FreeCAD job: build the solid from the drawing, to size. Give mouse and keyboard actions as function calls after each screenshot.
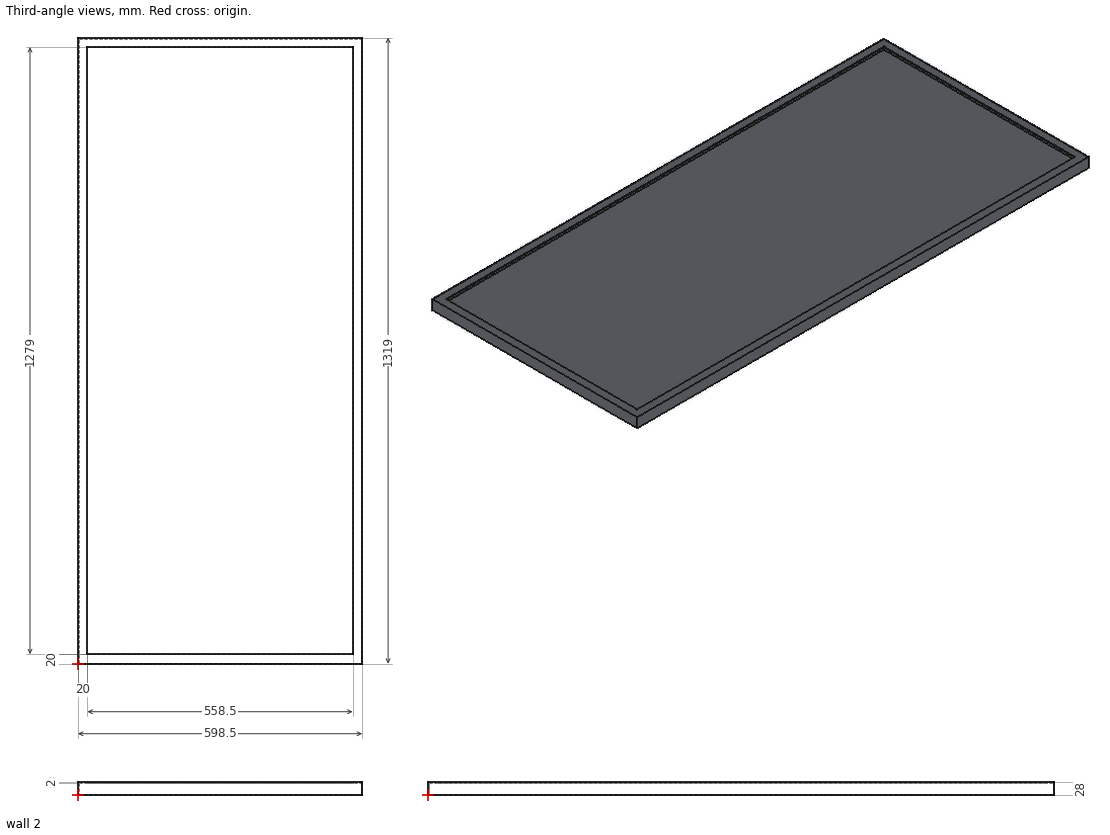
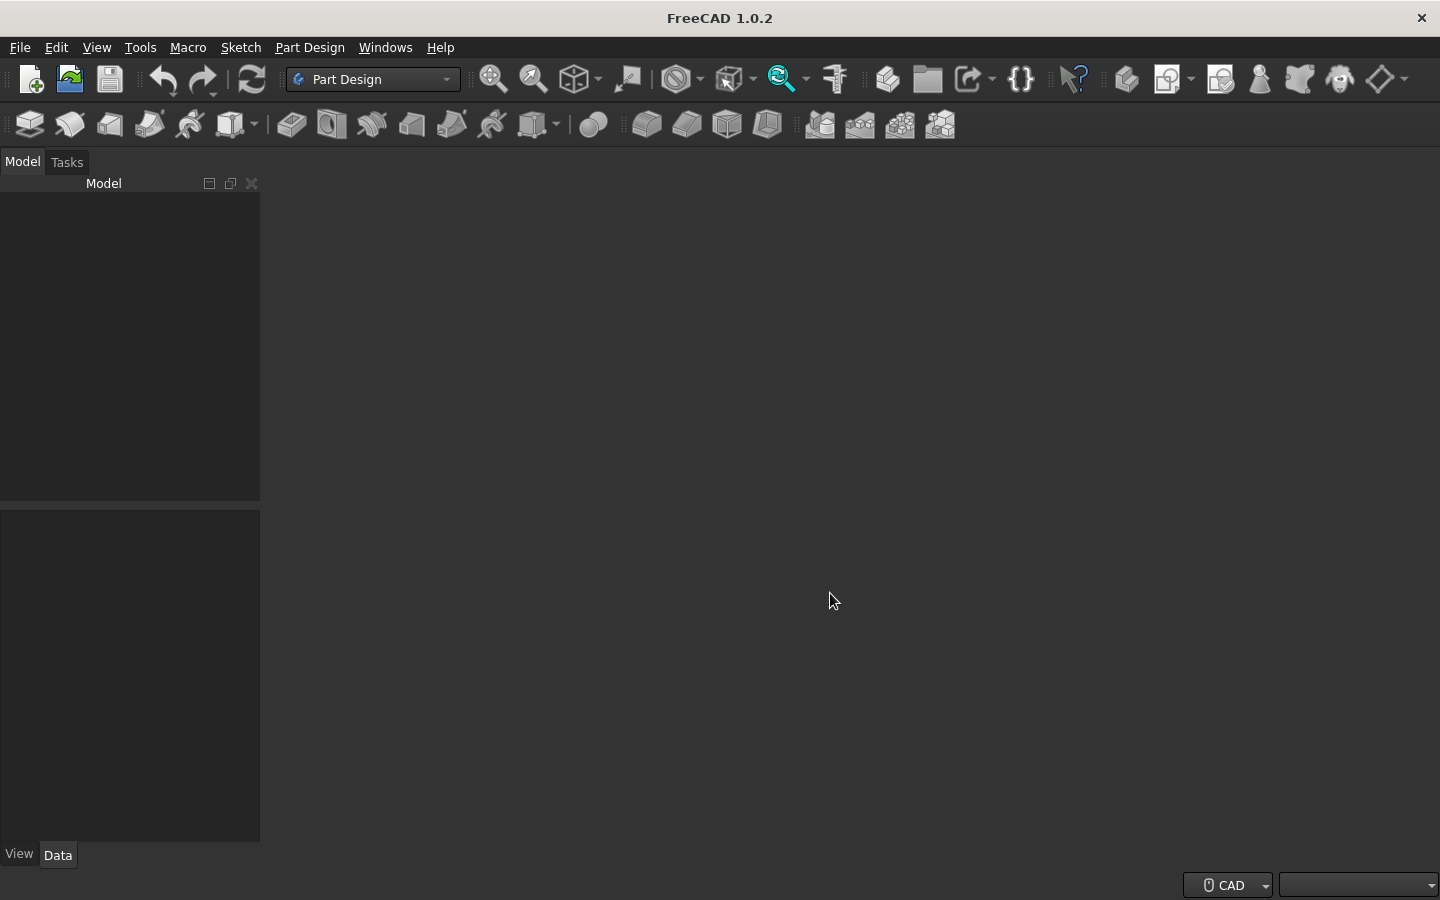
key(ctrl+n)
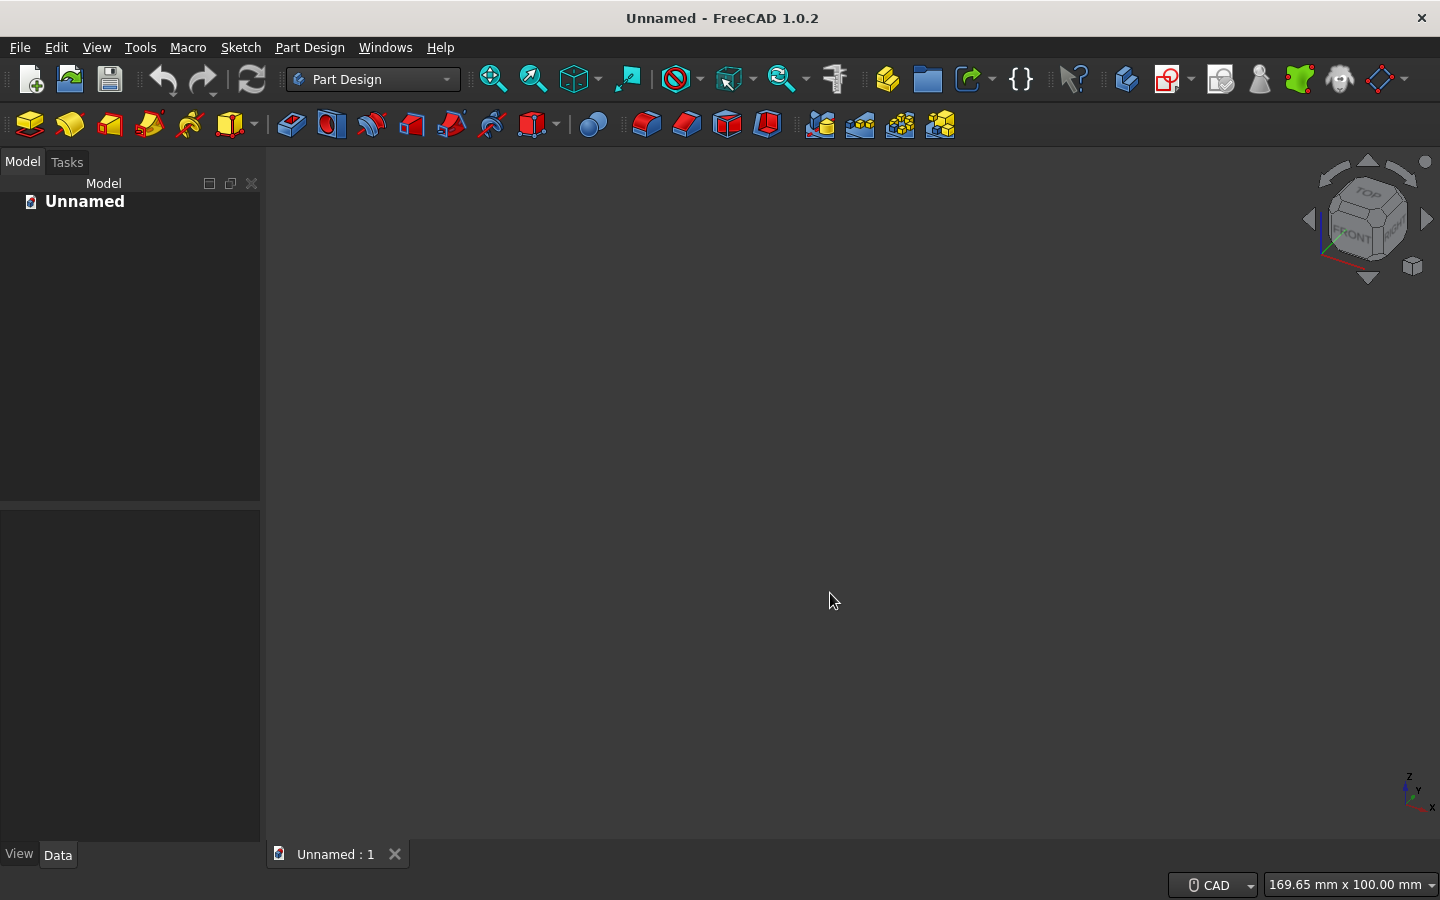
click(1168, 80)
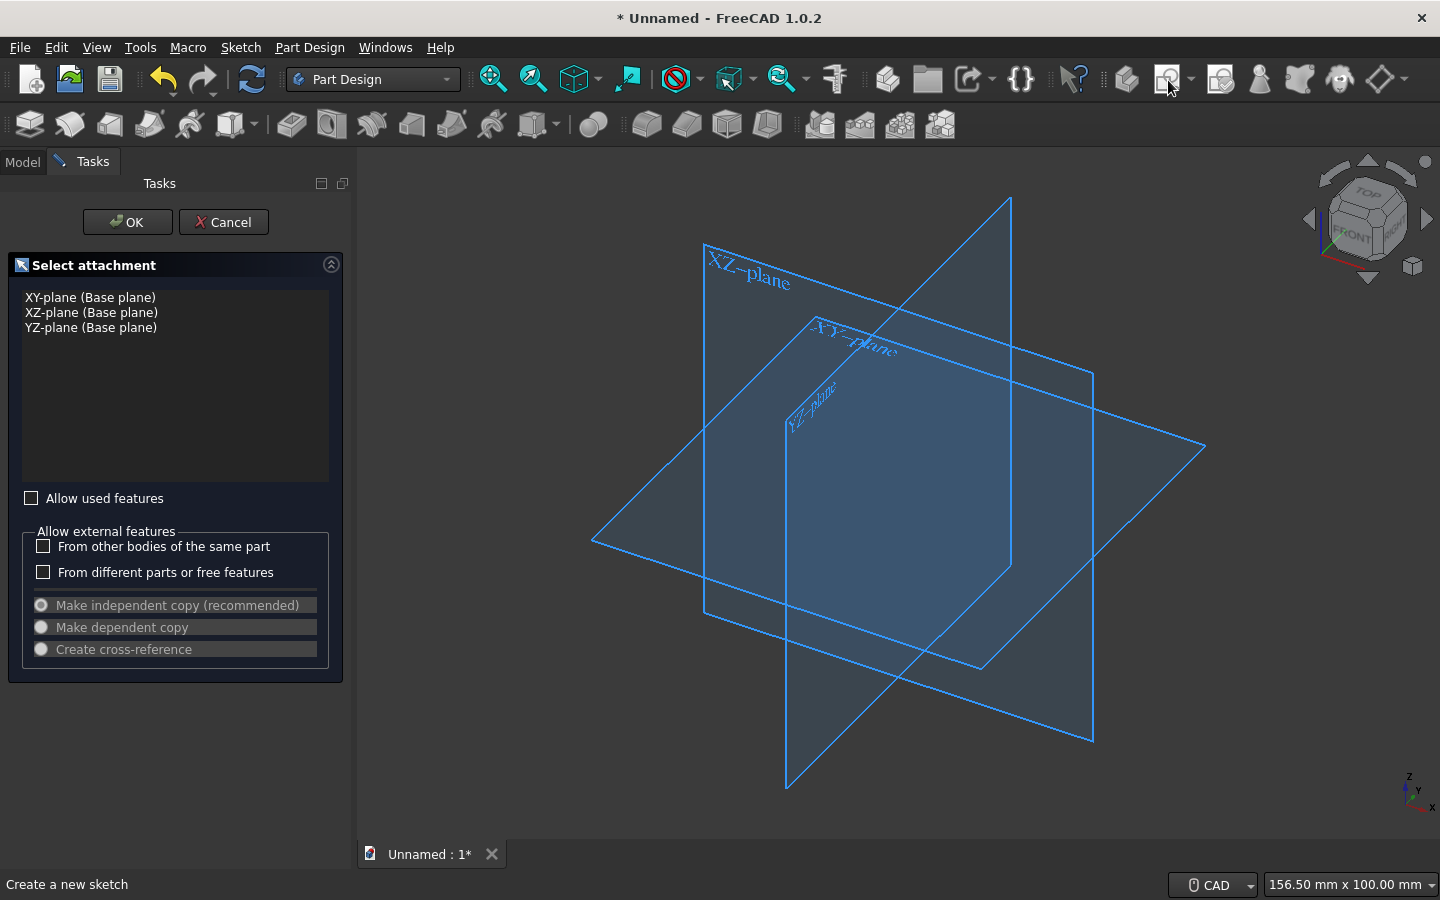
click(82, 298)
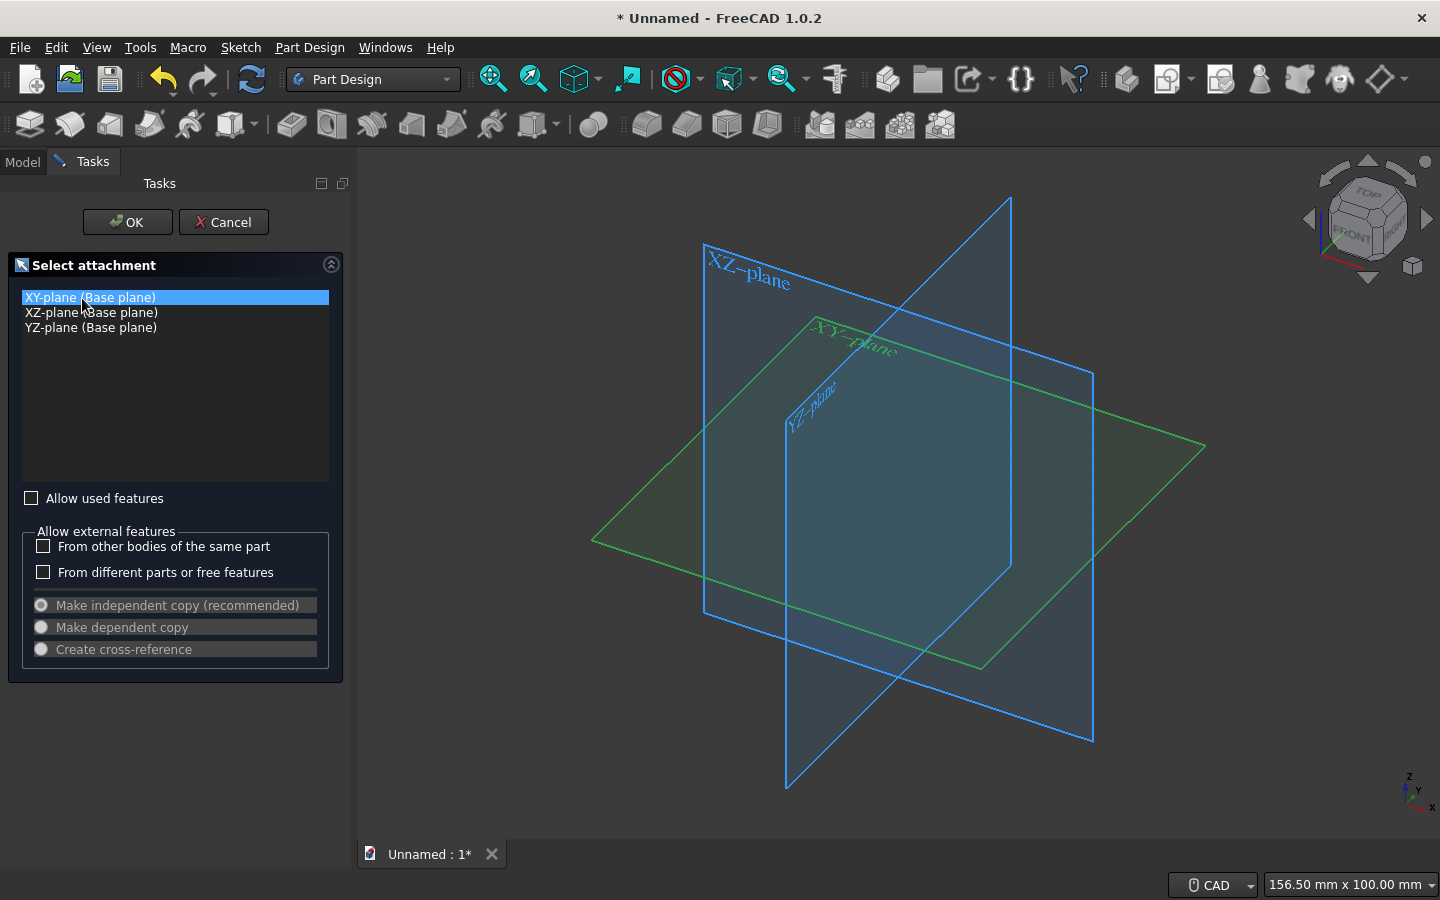
click(128, 222)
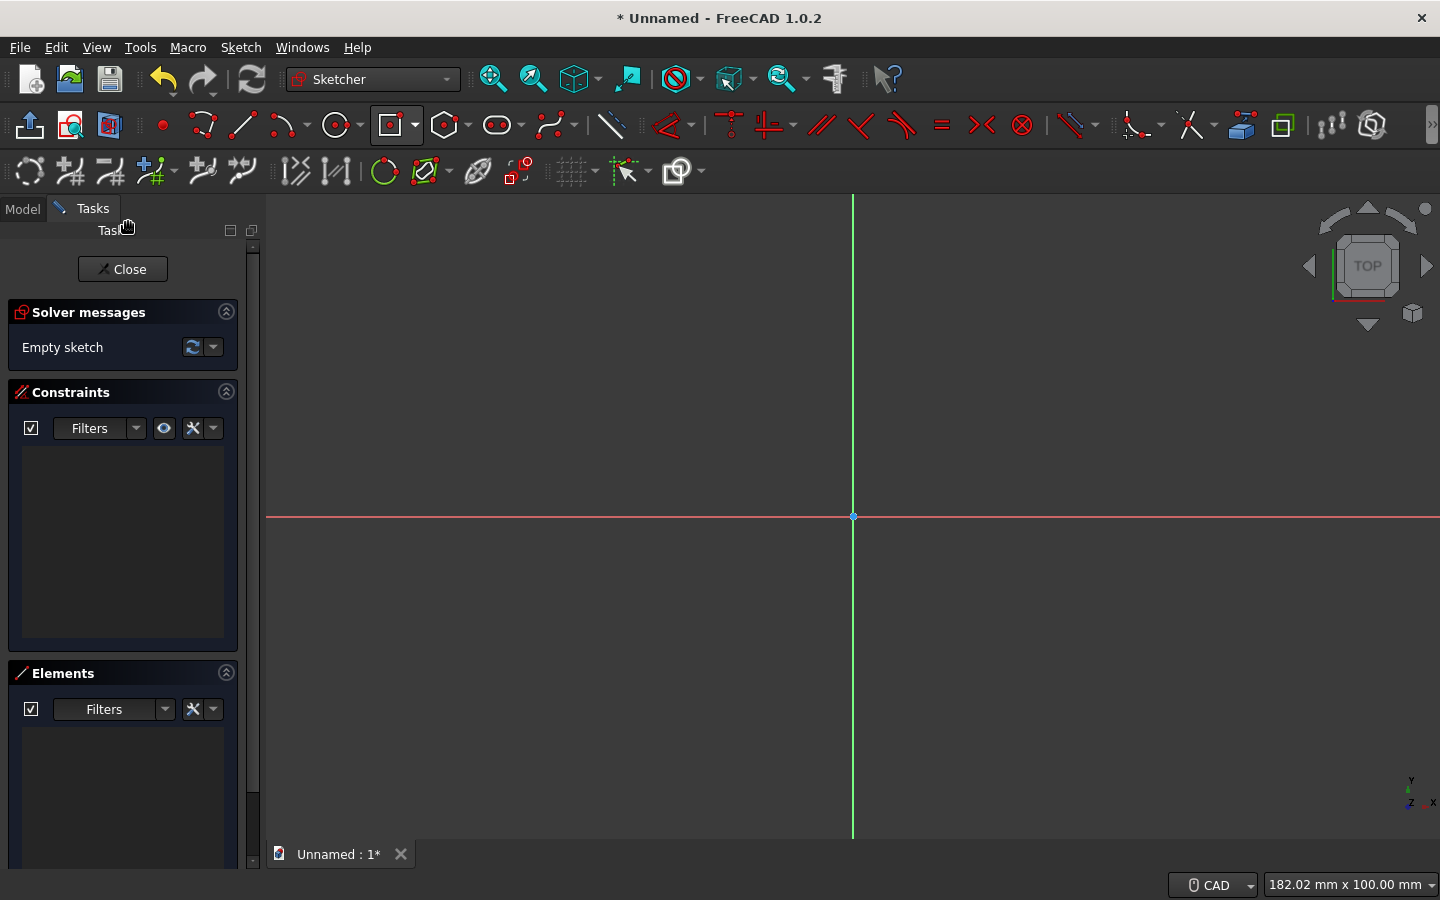
scroll(680, 739, down, 15)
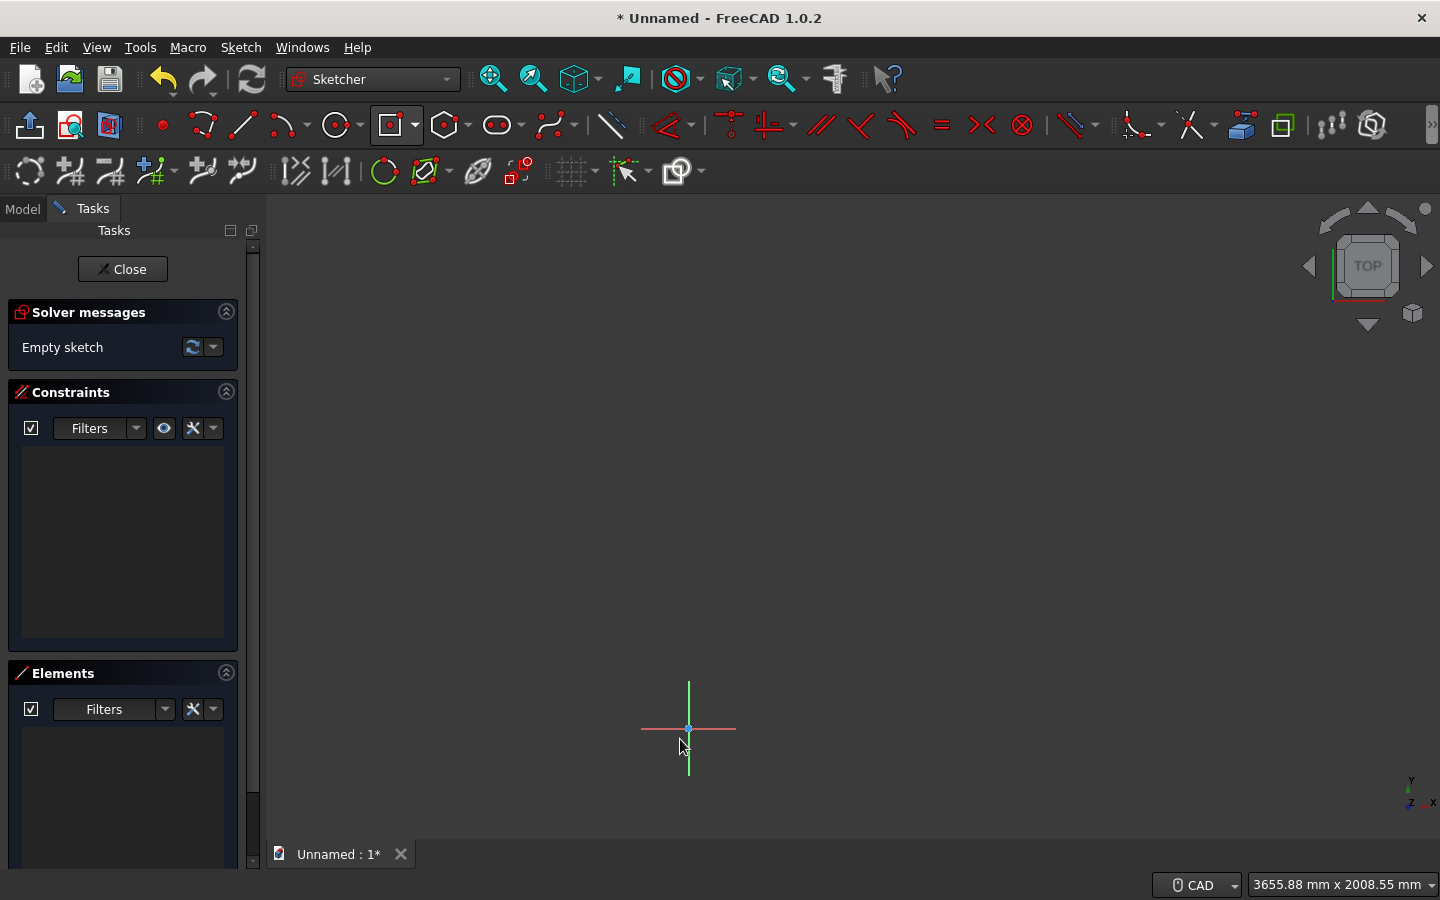
key(g)
key(r)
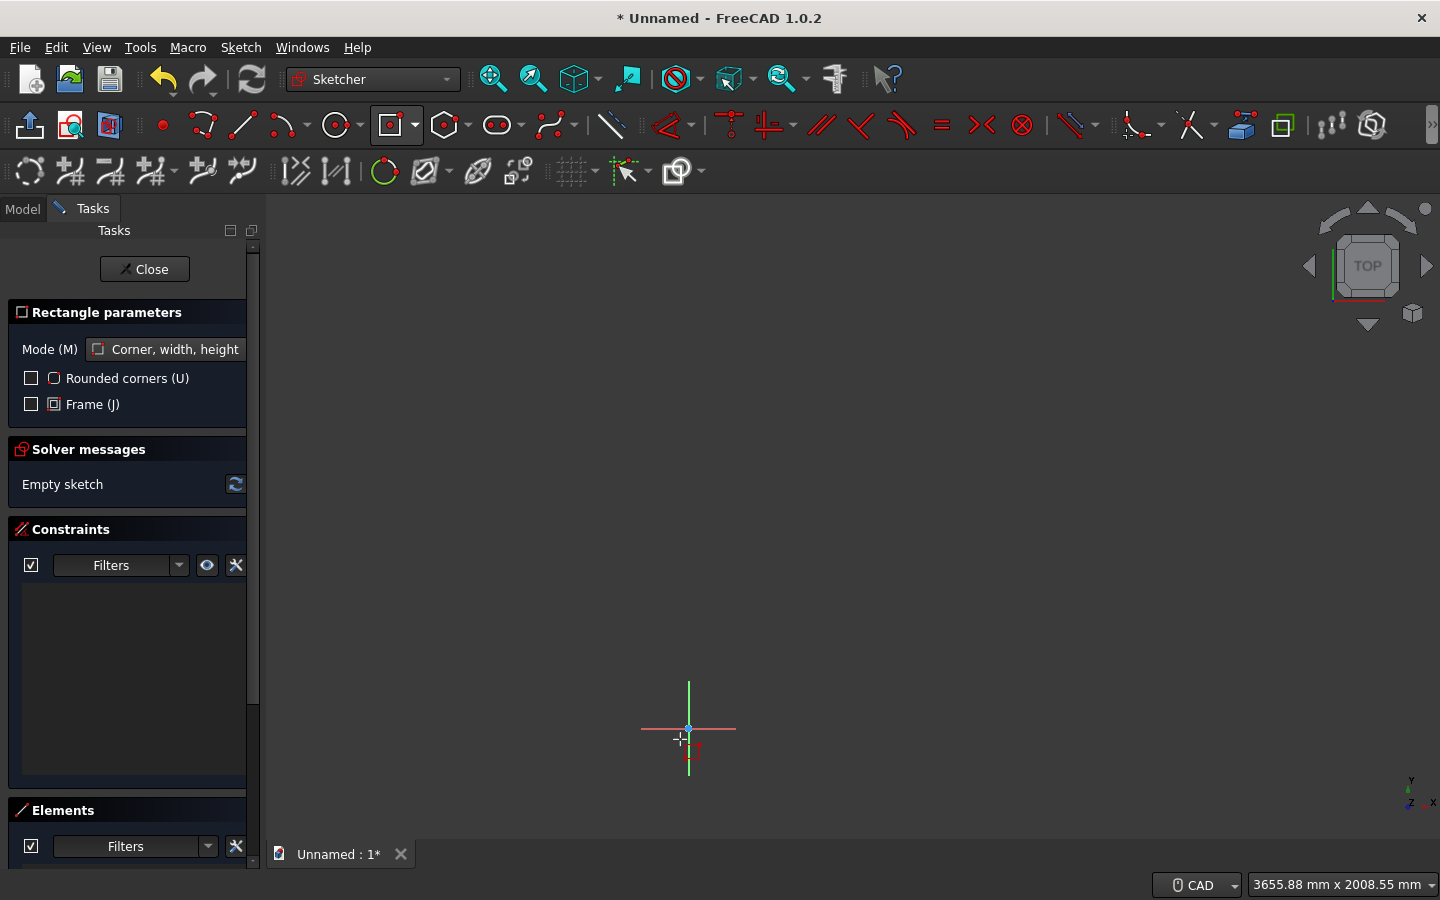
click(689, 729)
click(881, 305)
key(Escape)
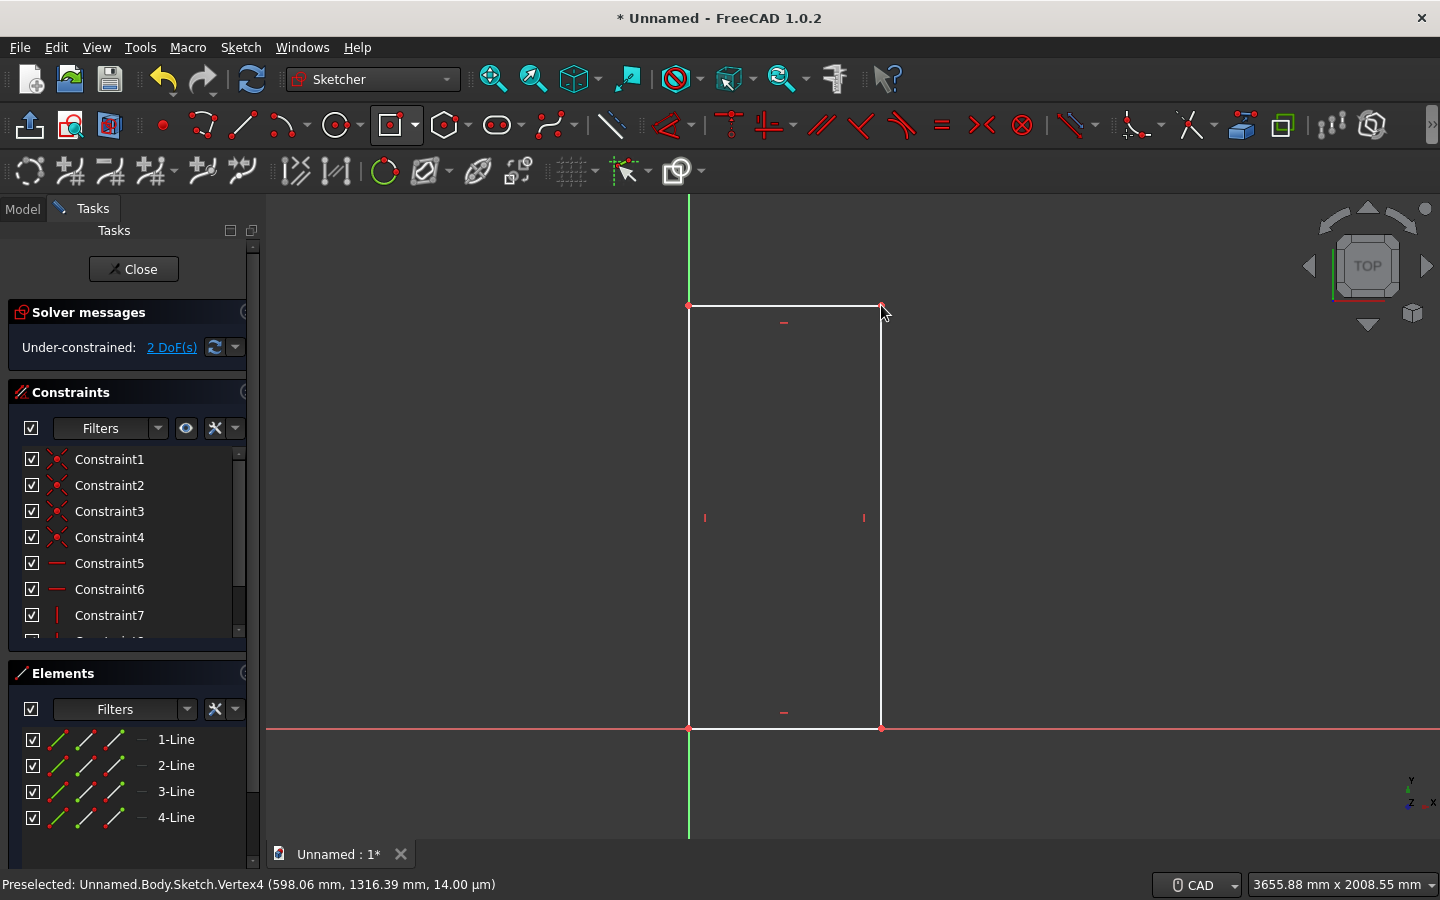
click(881, 602)